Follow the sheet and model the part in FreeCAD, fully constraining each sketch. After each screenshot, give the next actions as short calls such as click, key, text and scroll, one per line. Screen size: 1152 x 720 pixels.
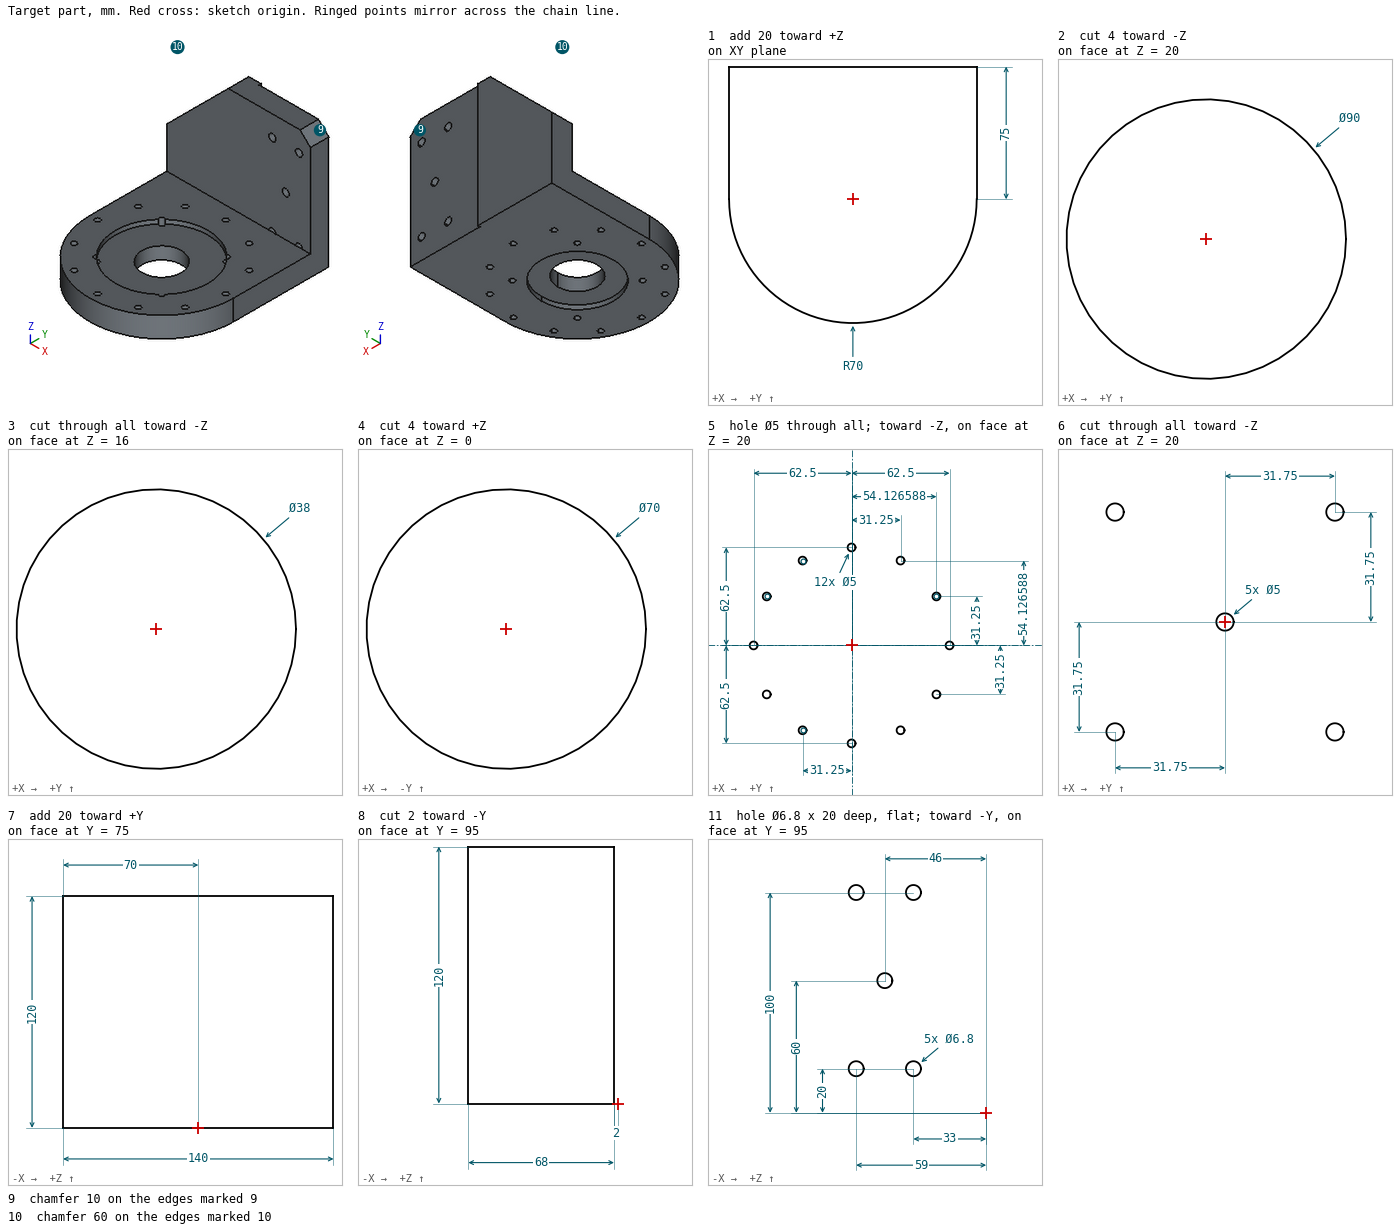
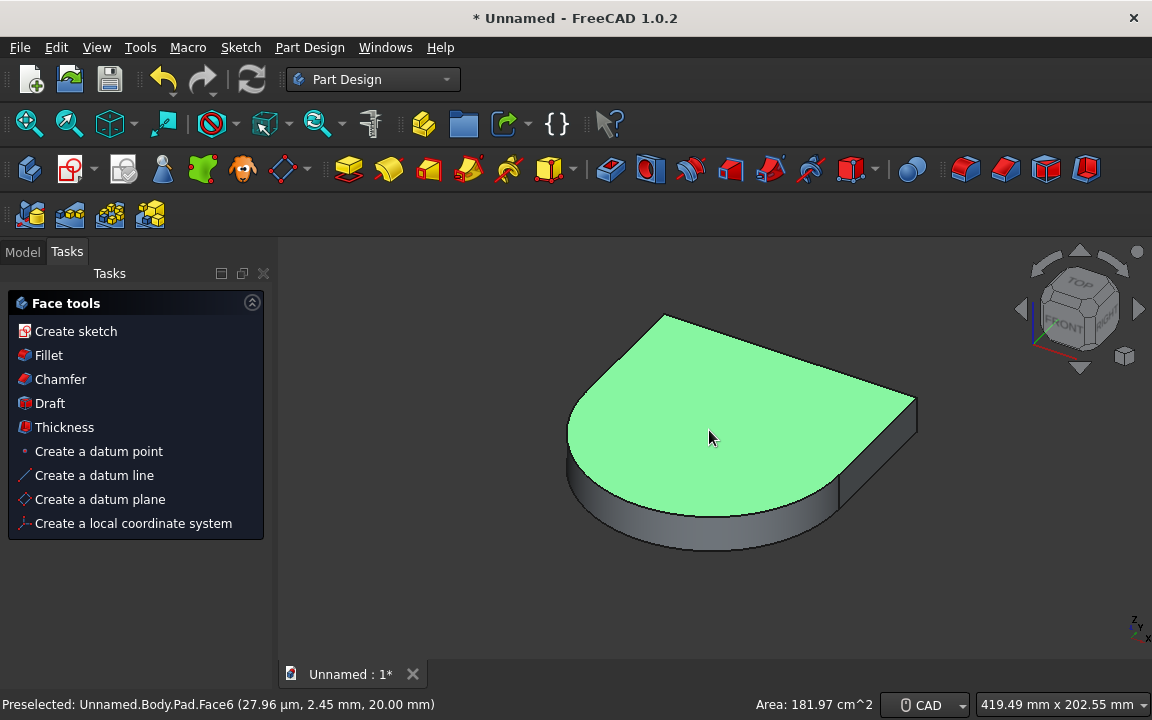
click(70, 170)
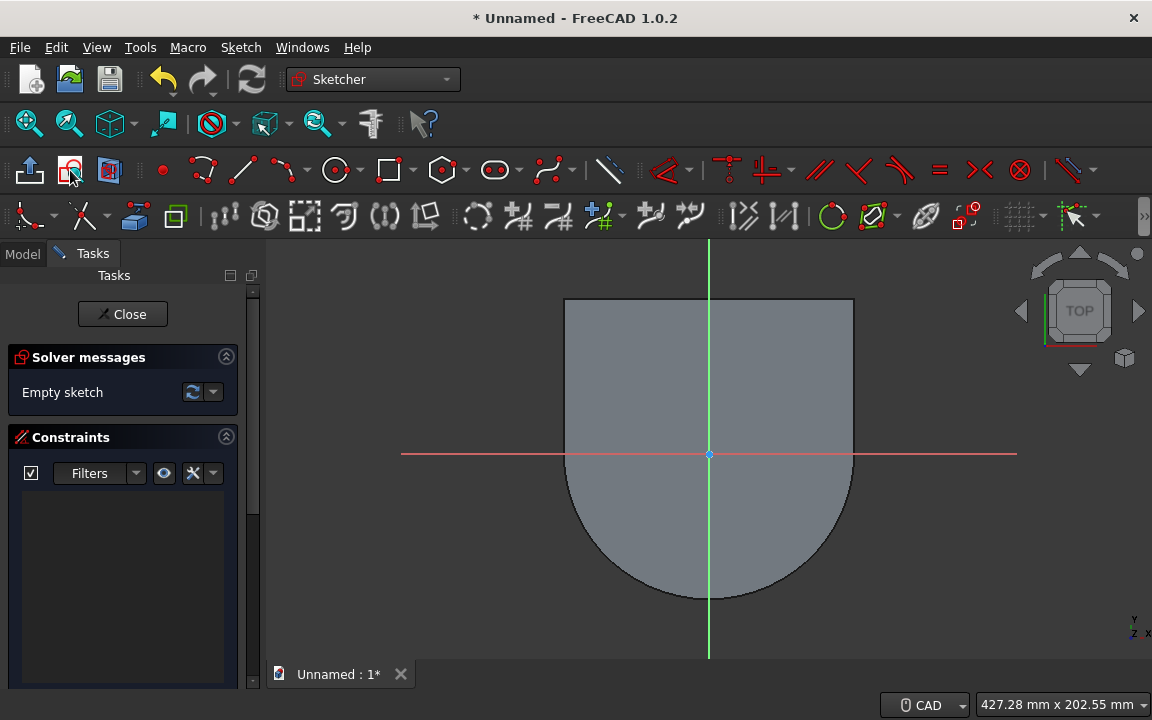
scroll(848, 465, up, 2)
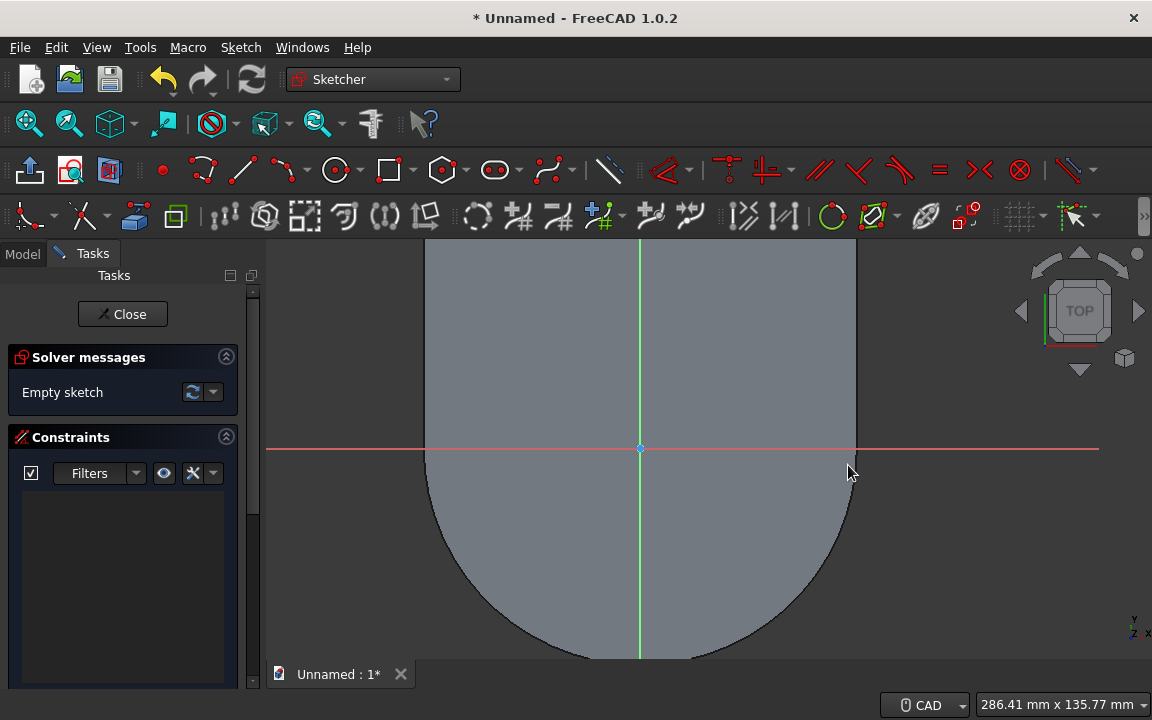
click(336, 170)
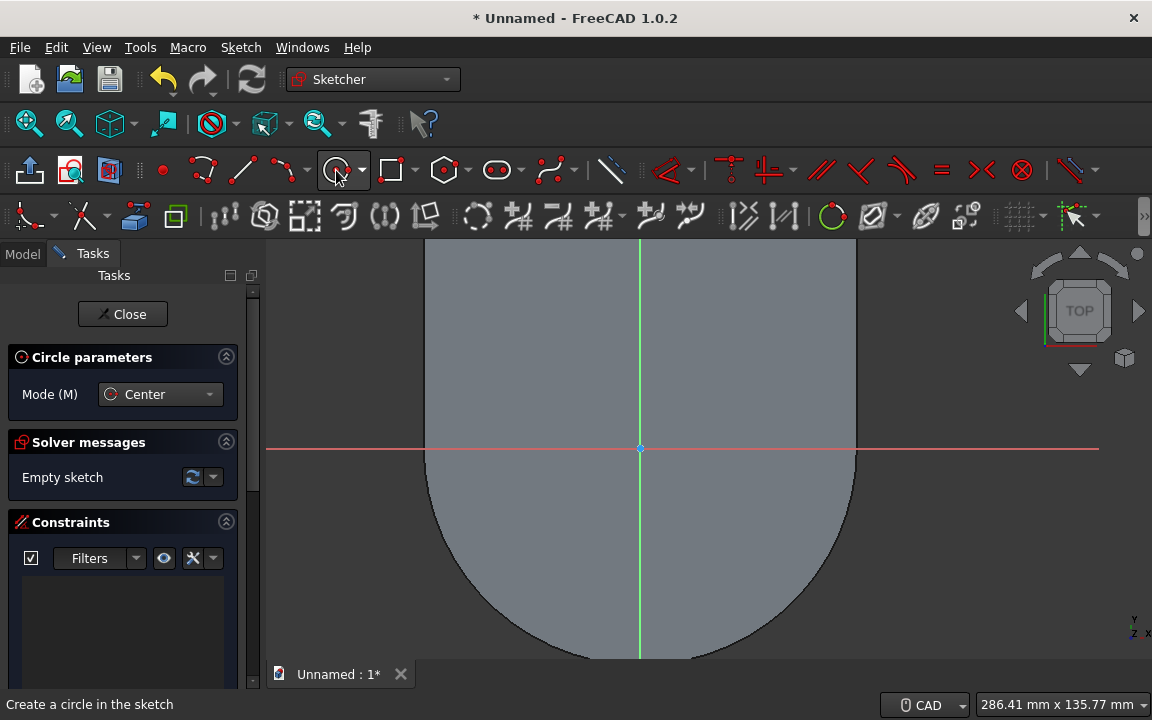
click(640, 449)
move(739, 350)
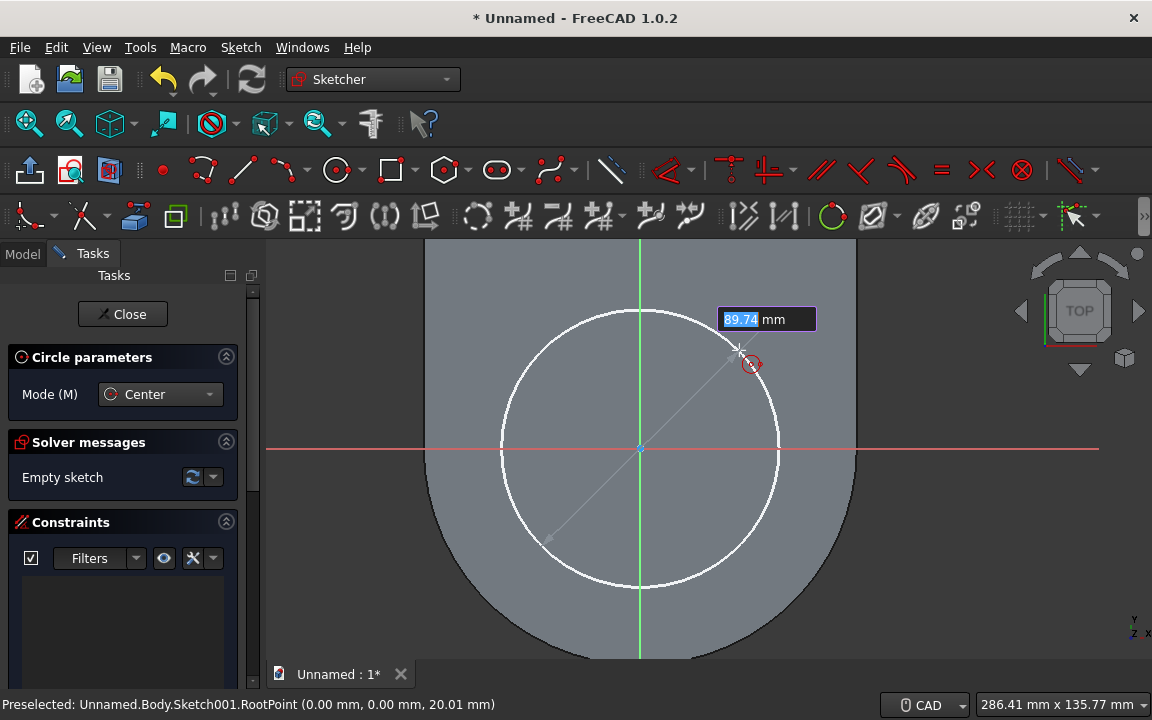
text(90)
key(Return)
key(Escape)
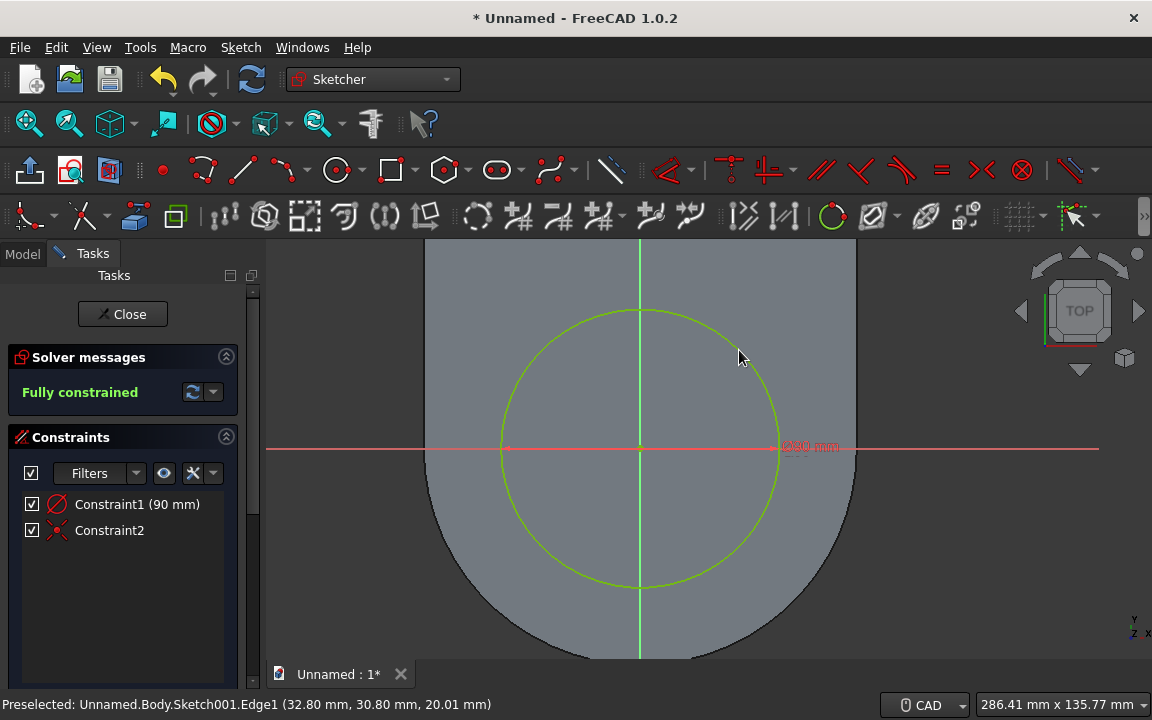
click(123, 314)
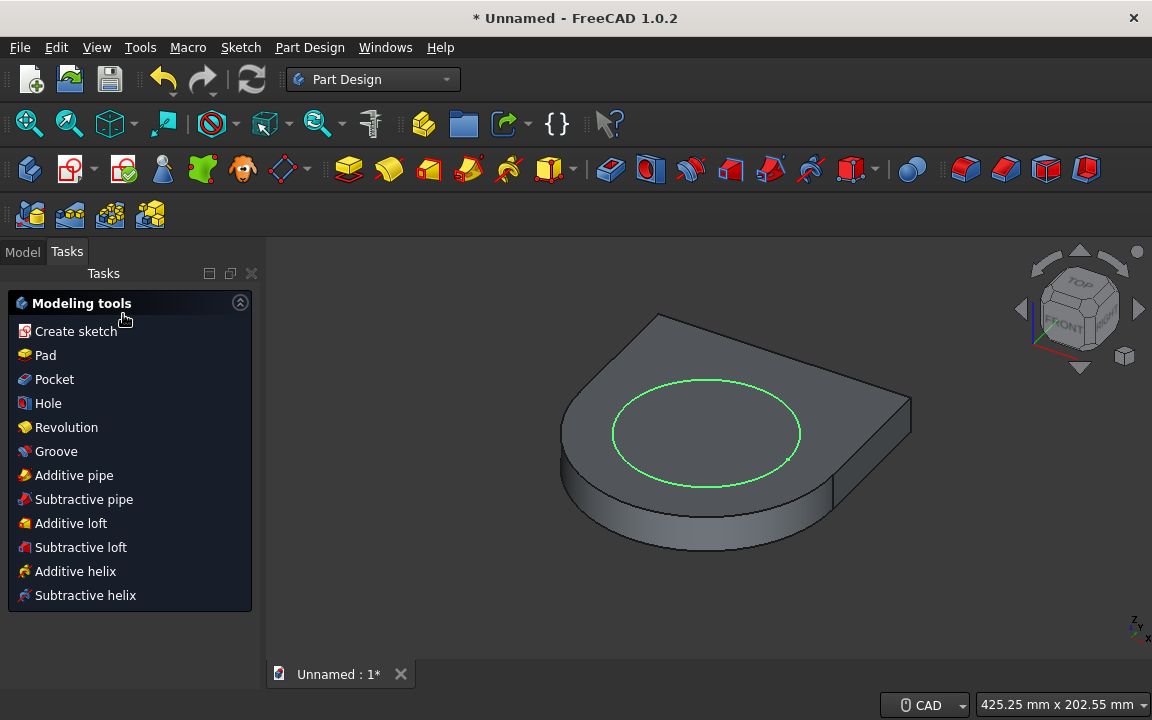
click(612, 170)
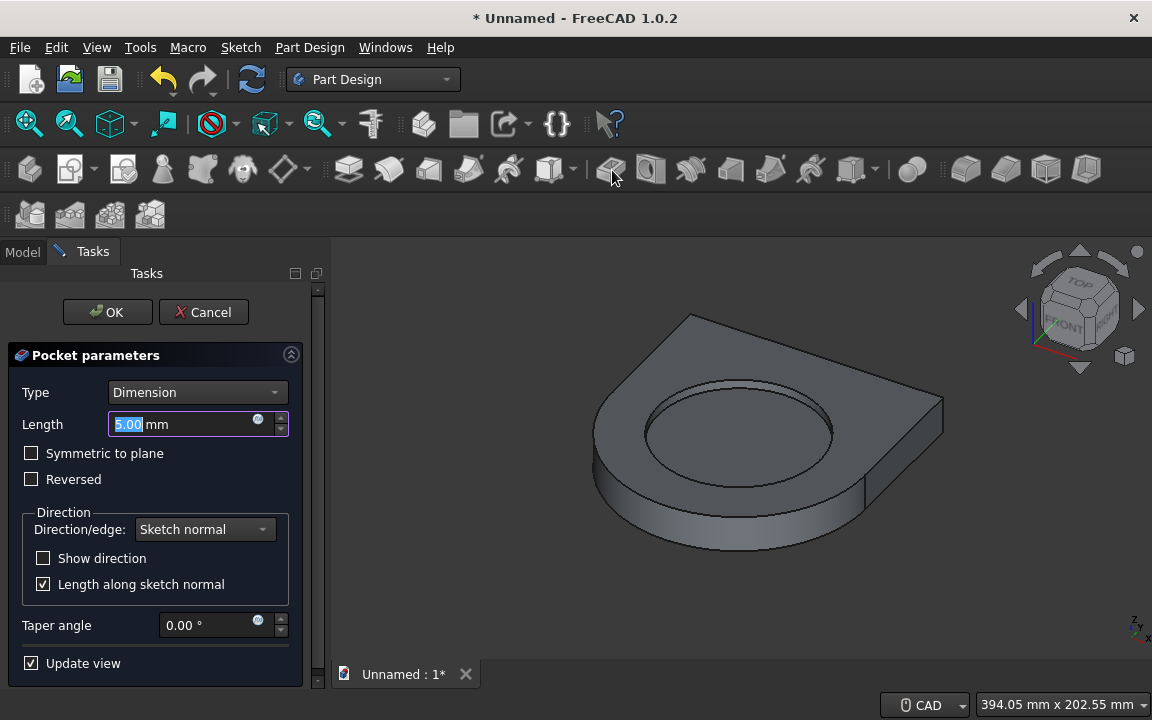
text(4)
key(Tab)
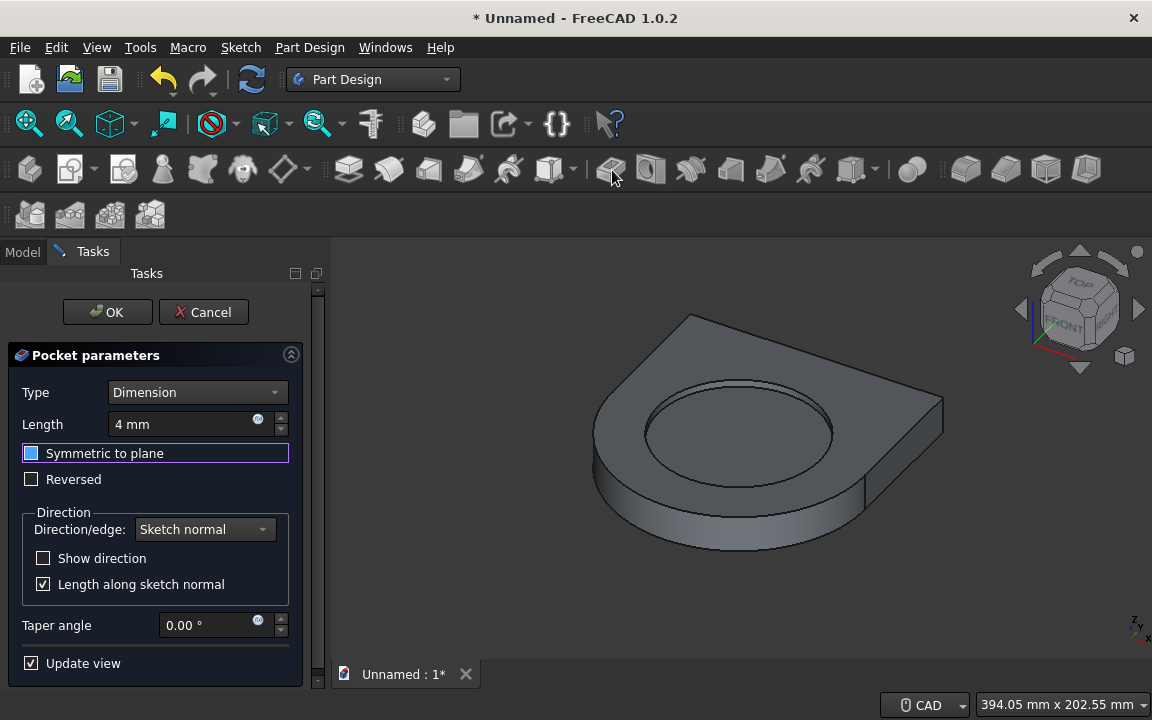
click(108, 312)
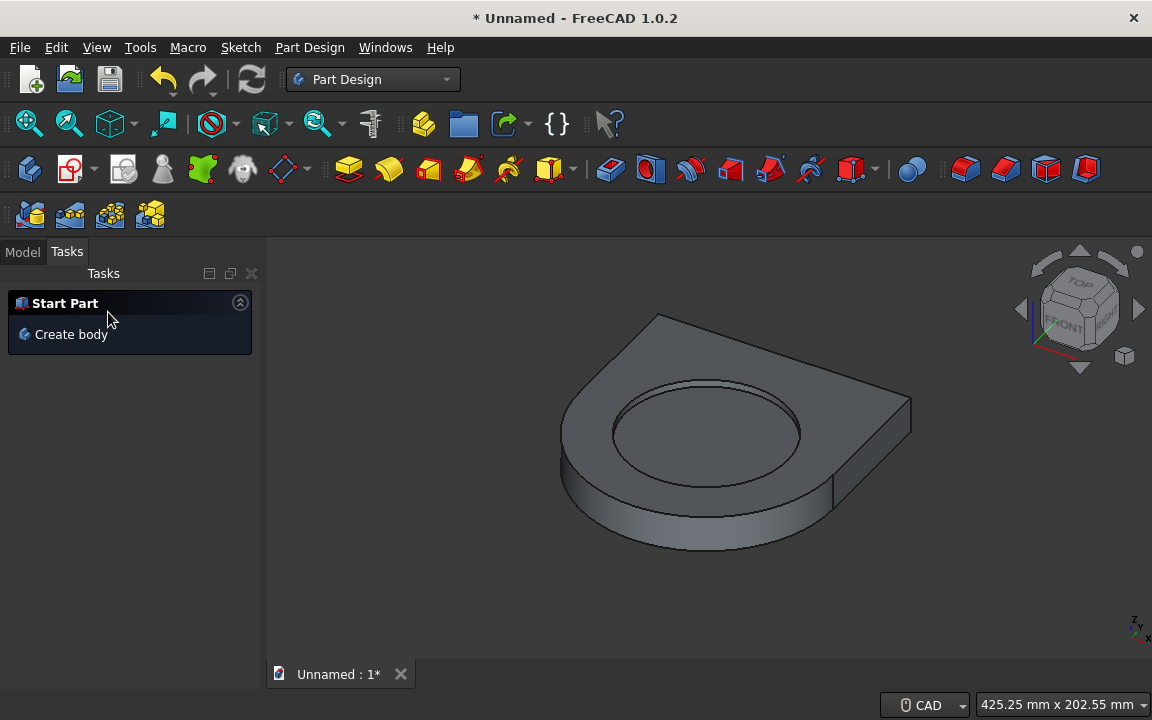
click(706, 439)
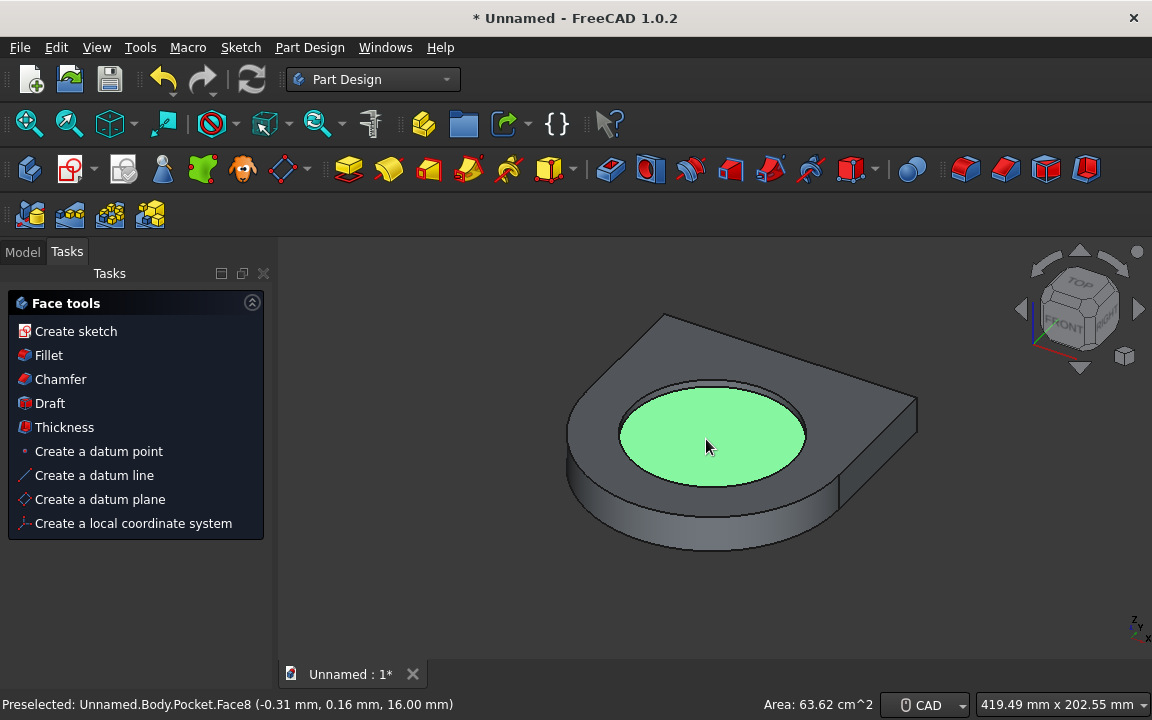
click(70, 170)